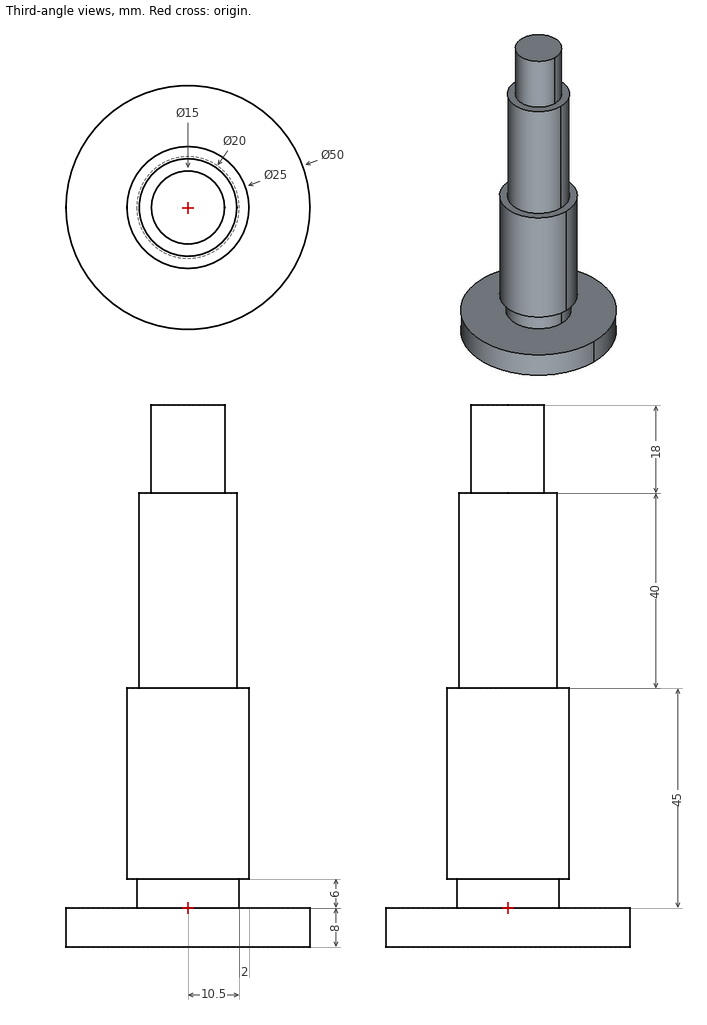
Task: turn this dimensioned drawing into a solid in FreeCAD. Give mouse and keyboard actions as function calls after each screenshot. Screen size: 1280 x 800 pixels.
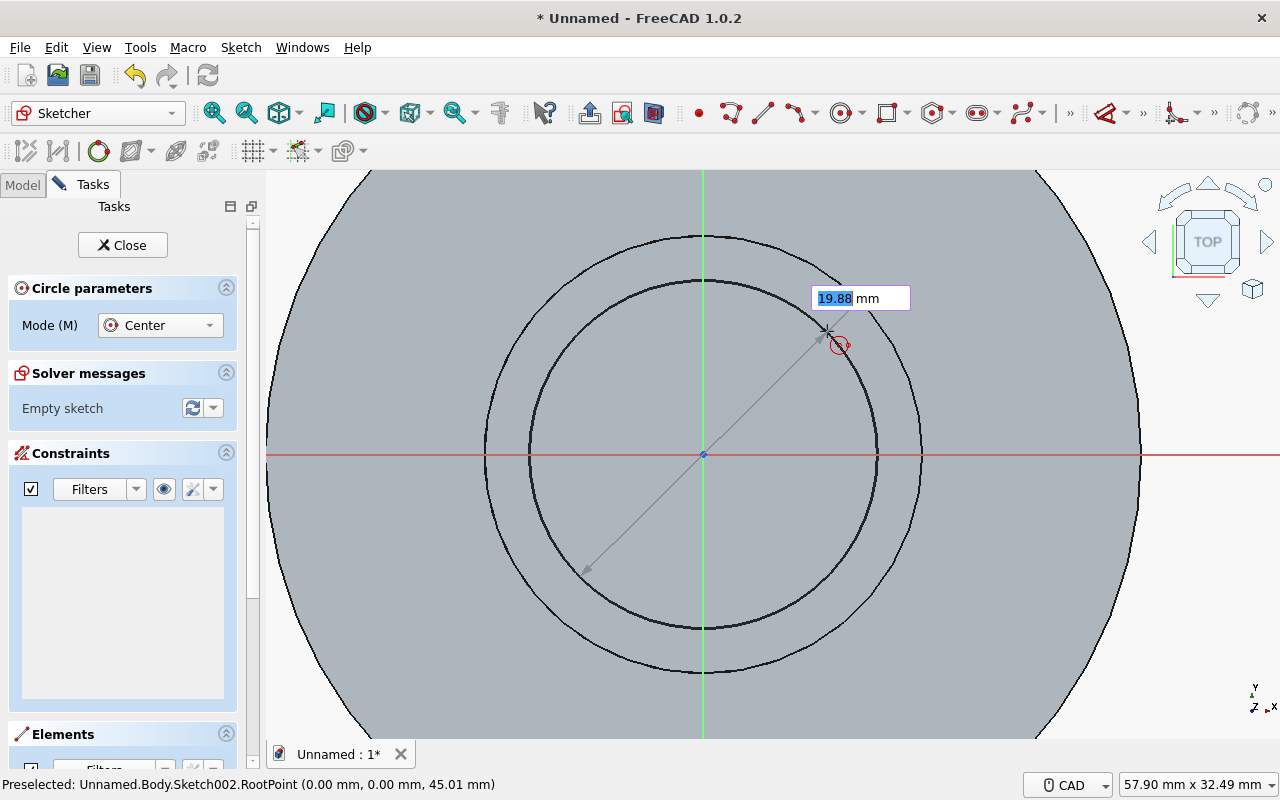
text(20)
key(Return)
key(Escape)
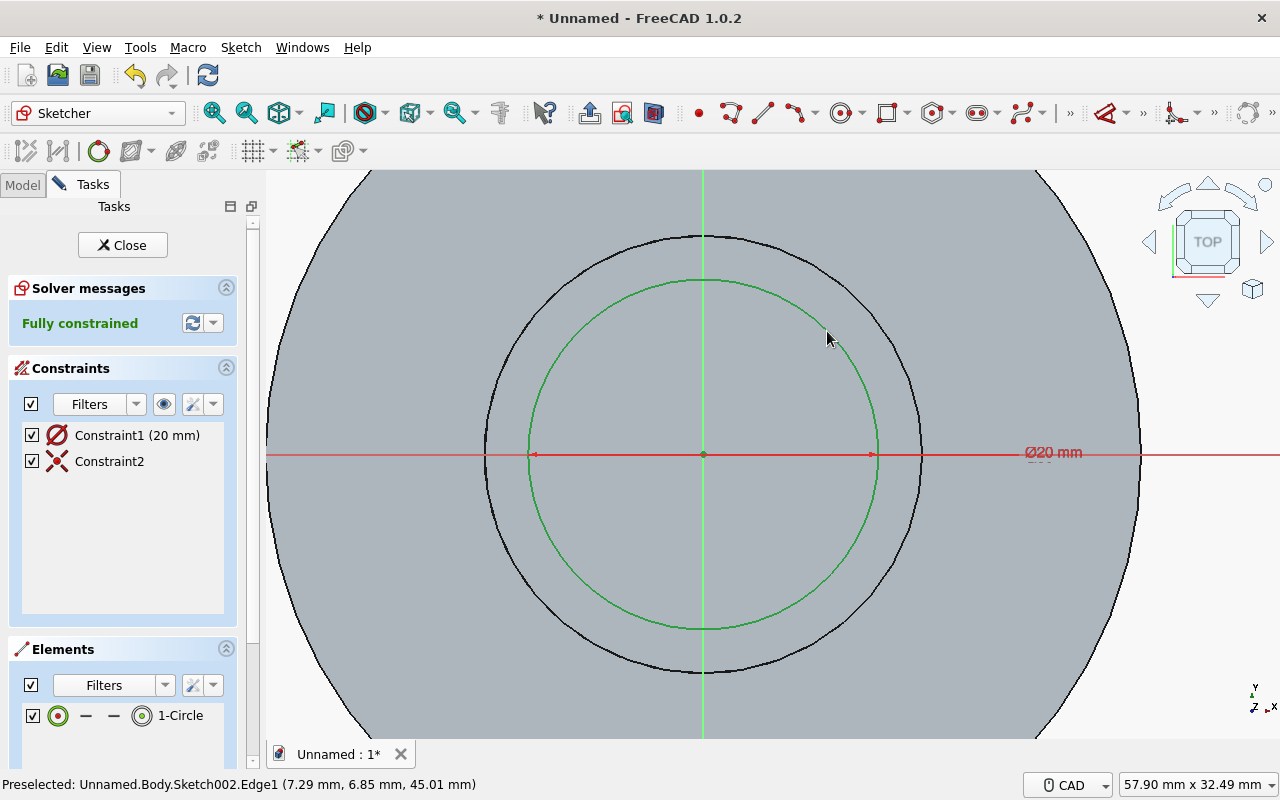
click(123, 245)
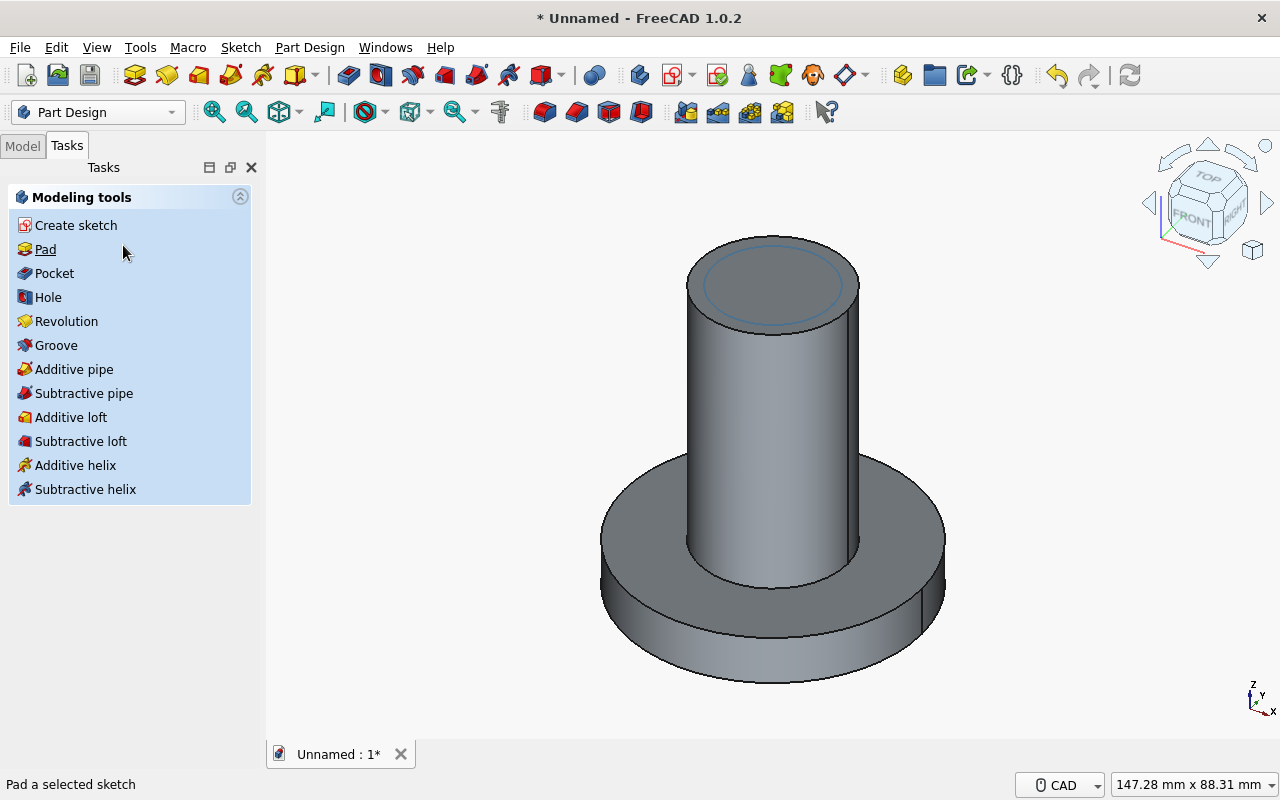
click(136, 76)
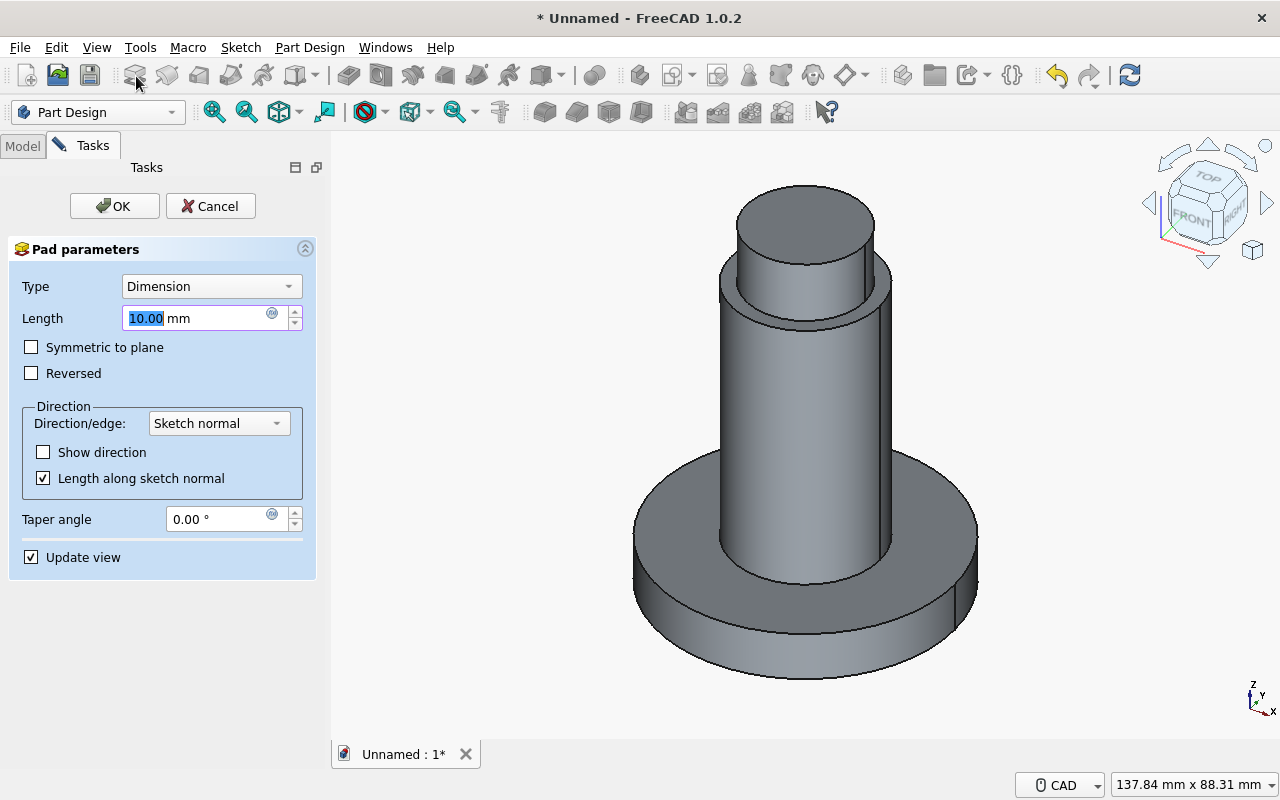
text(40)
key(Tab)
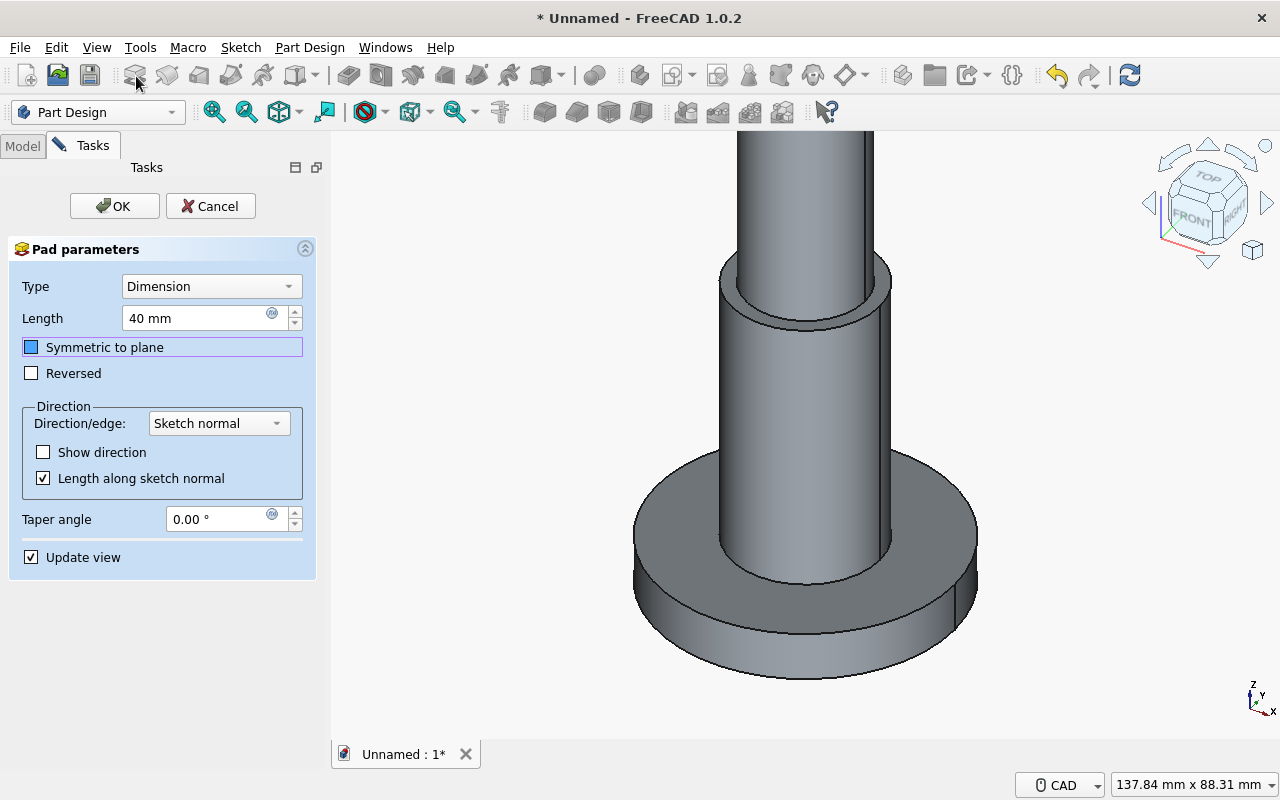
click(115, 206)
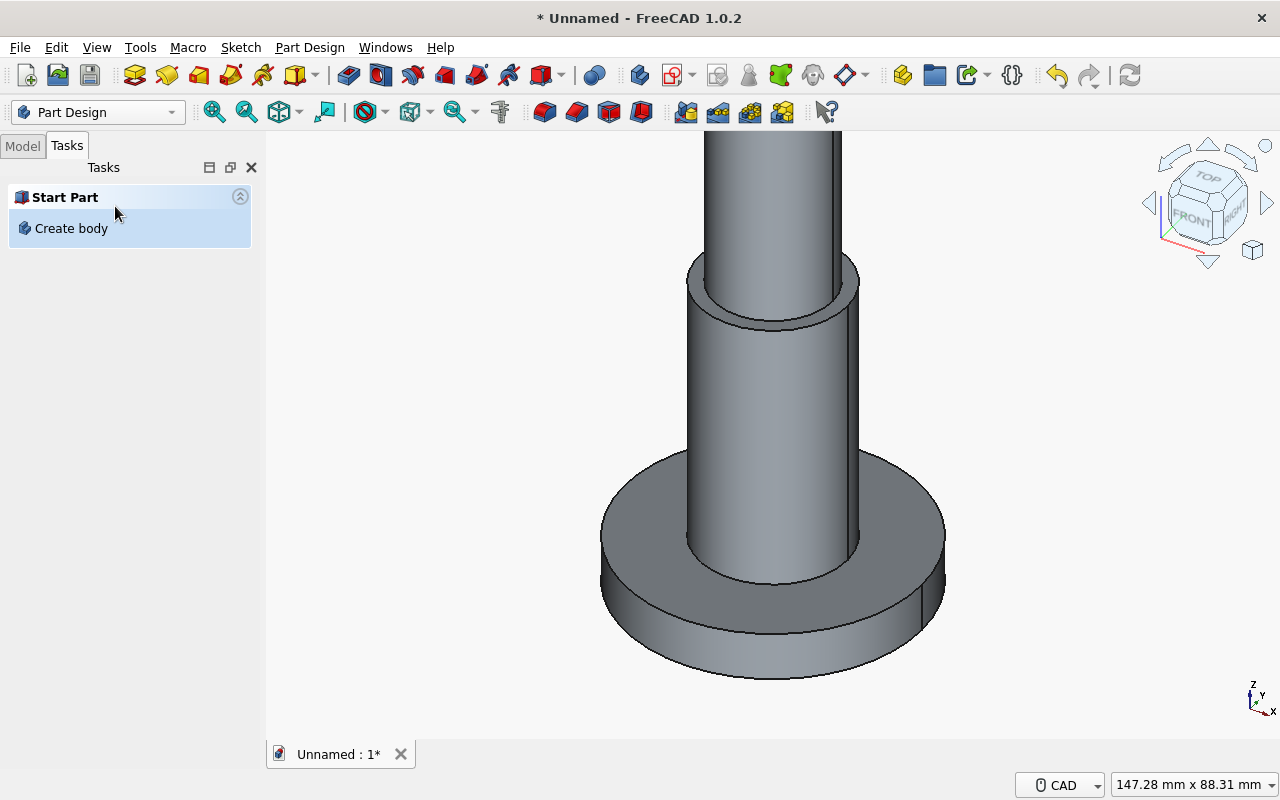
click(216, 112)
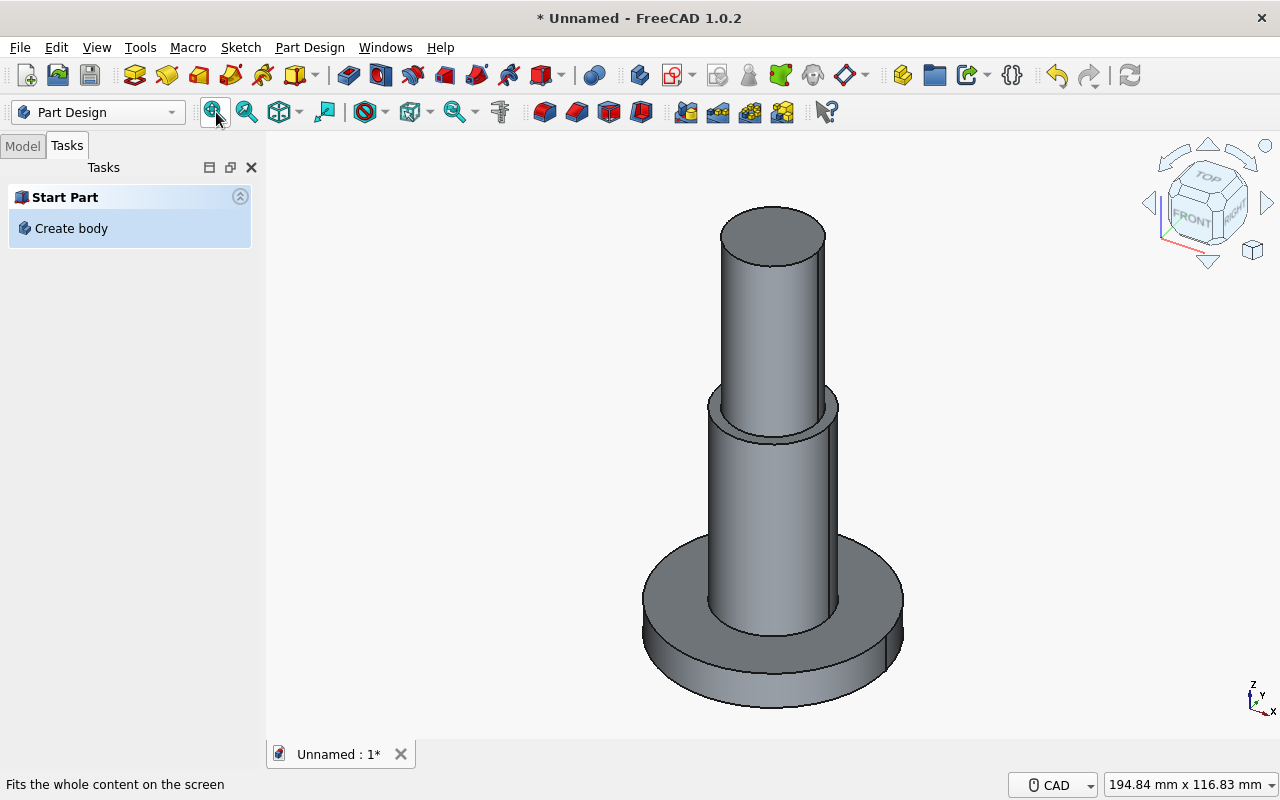
click(672, 76)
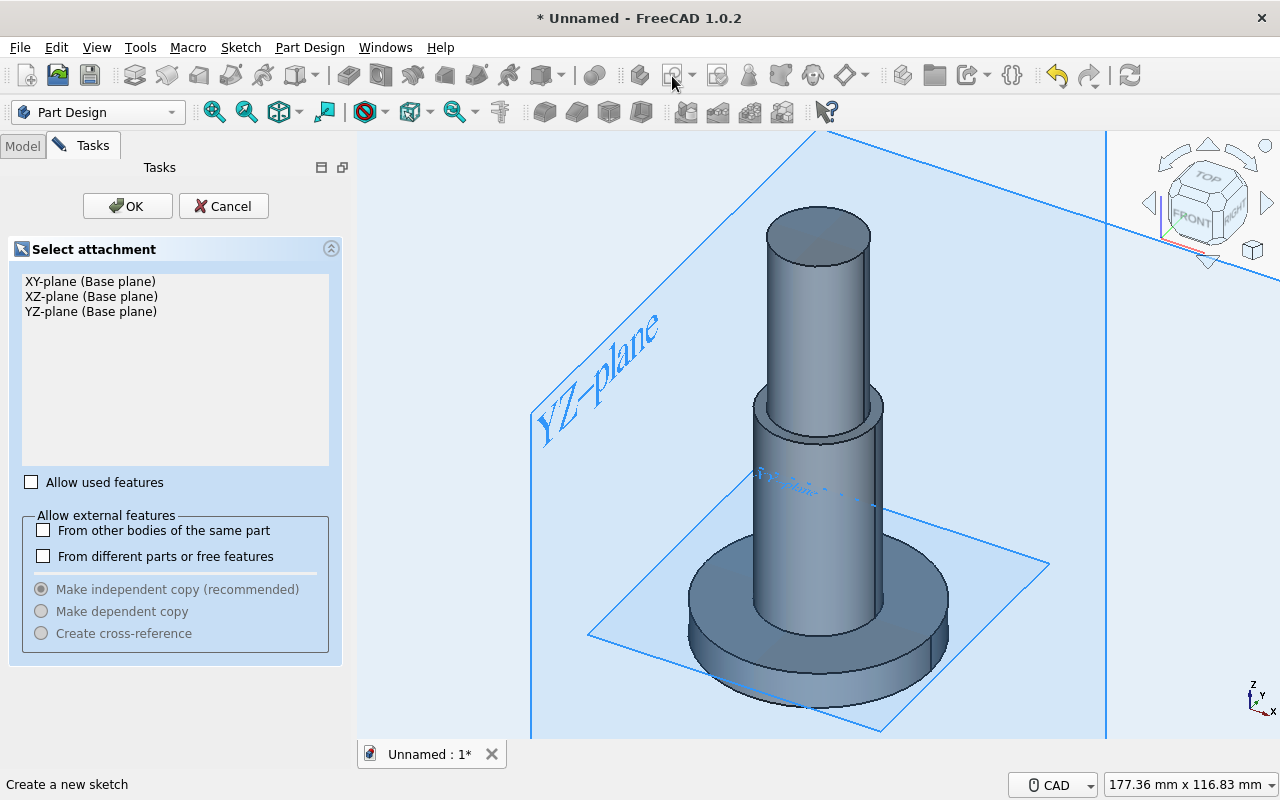
click(82, 296)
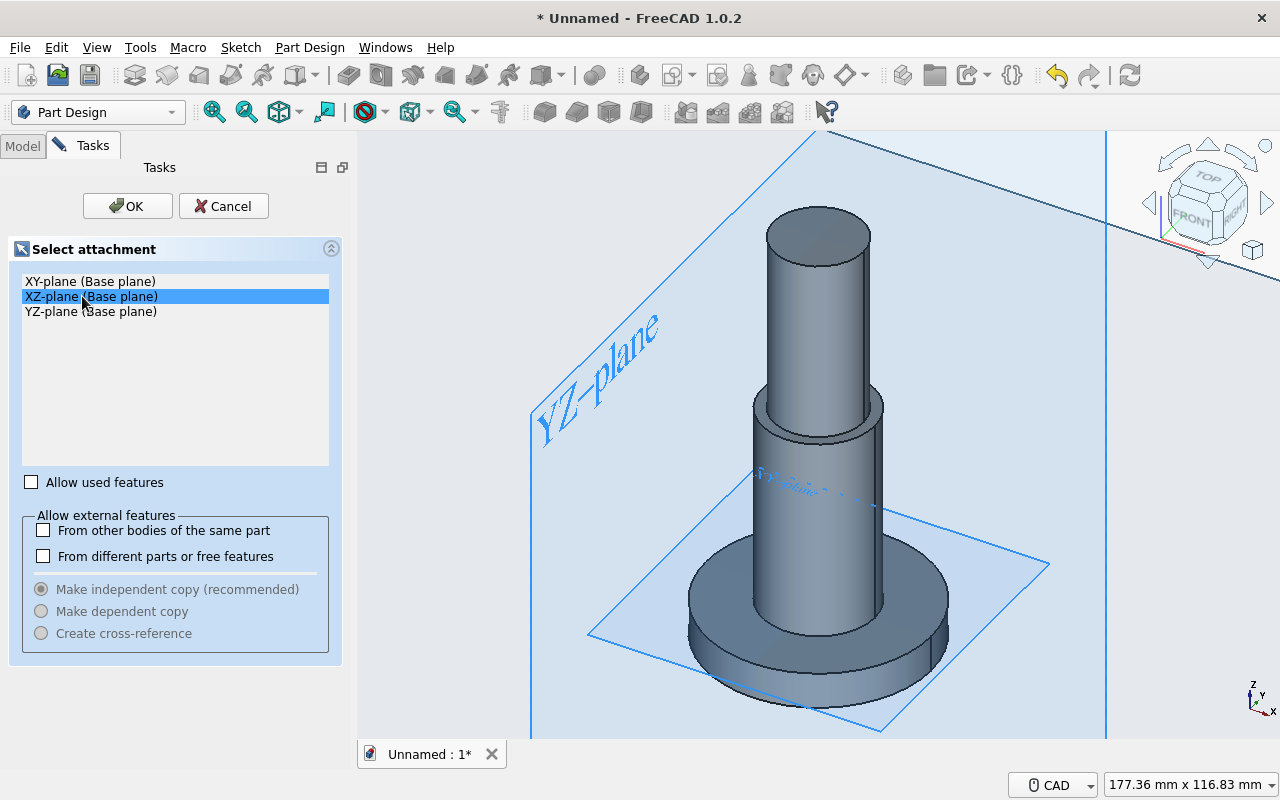
click(128, 206)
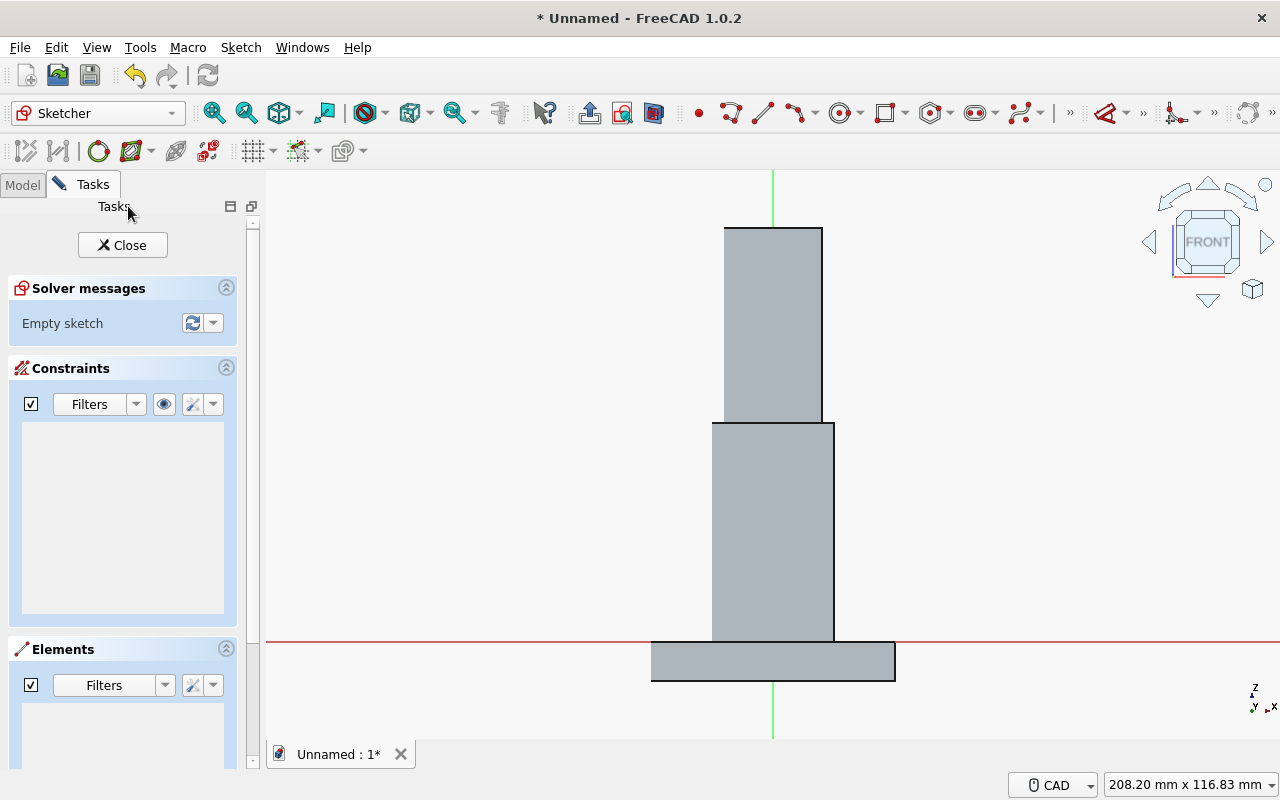
key(q)
key(s)